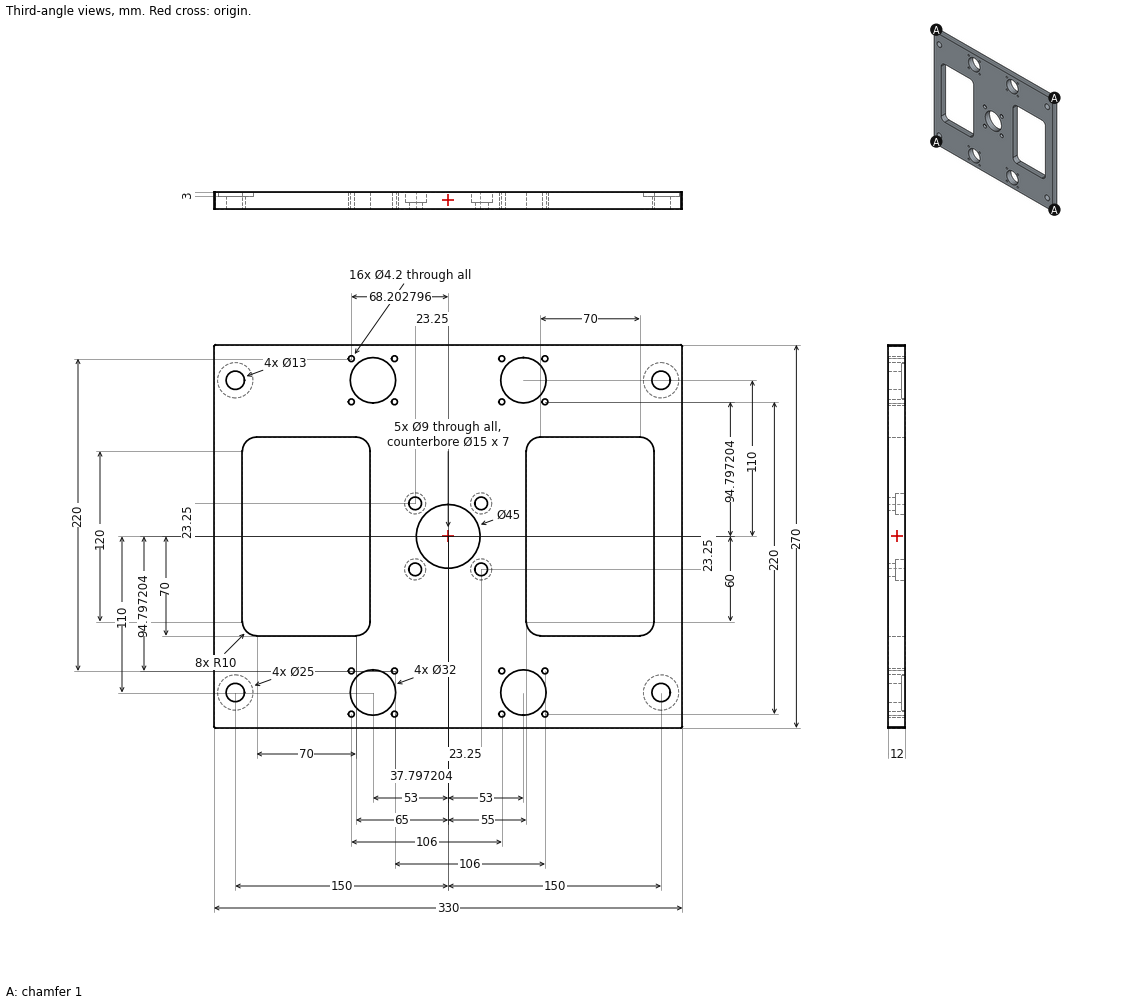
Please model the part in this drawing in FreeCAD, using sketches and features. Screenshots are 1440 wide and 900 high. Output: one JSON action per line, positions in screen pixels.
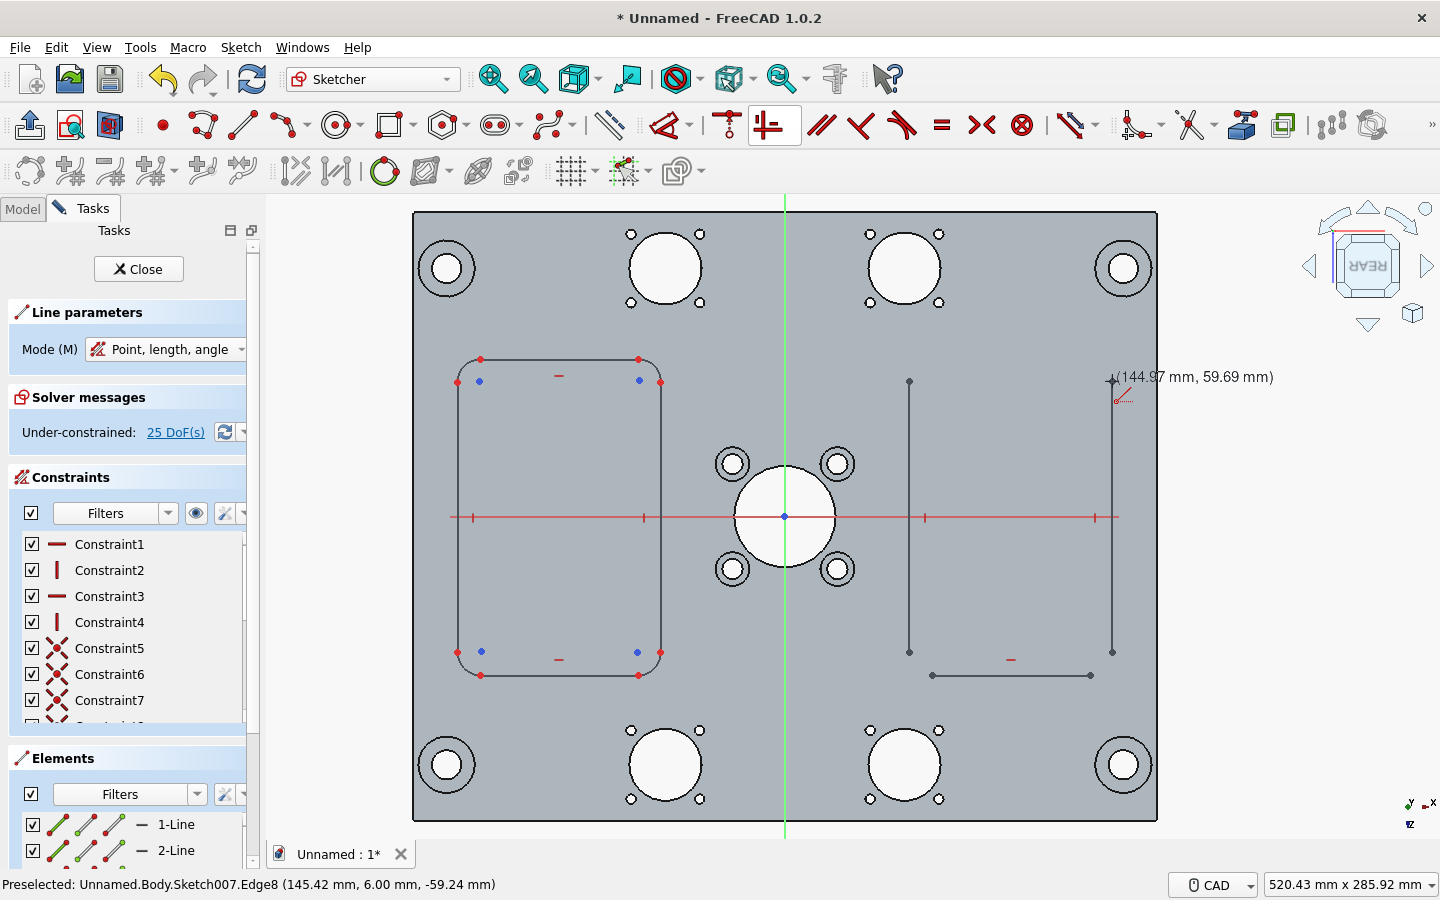
{"action": "left_click", "coordinate": [1090, 359]}
{"action": "left_click", "coordinate": [932, 359]}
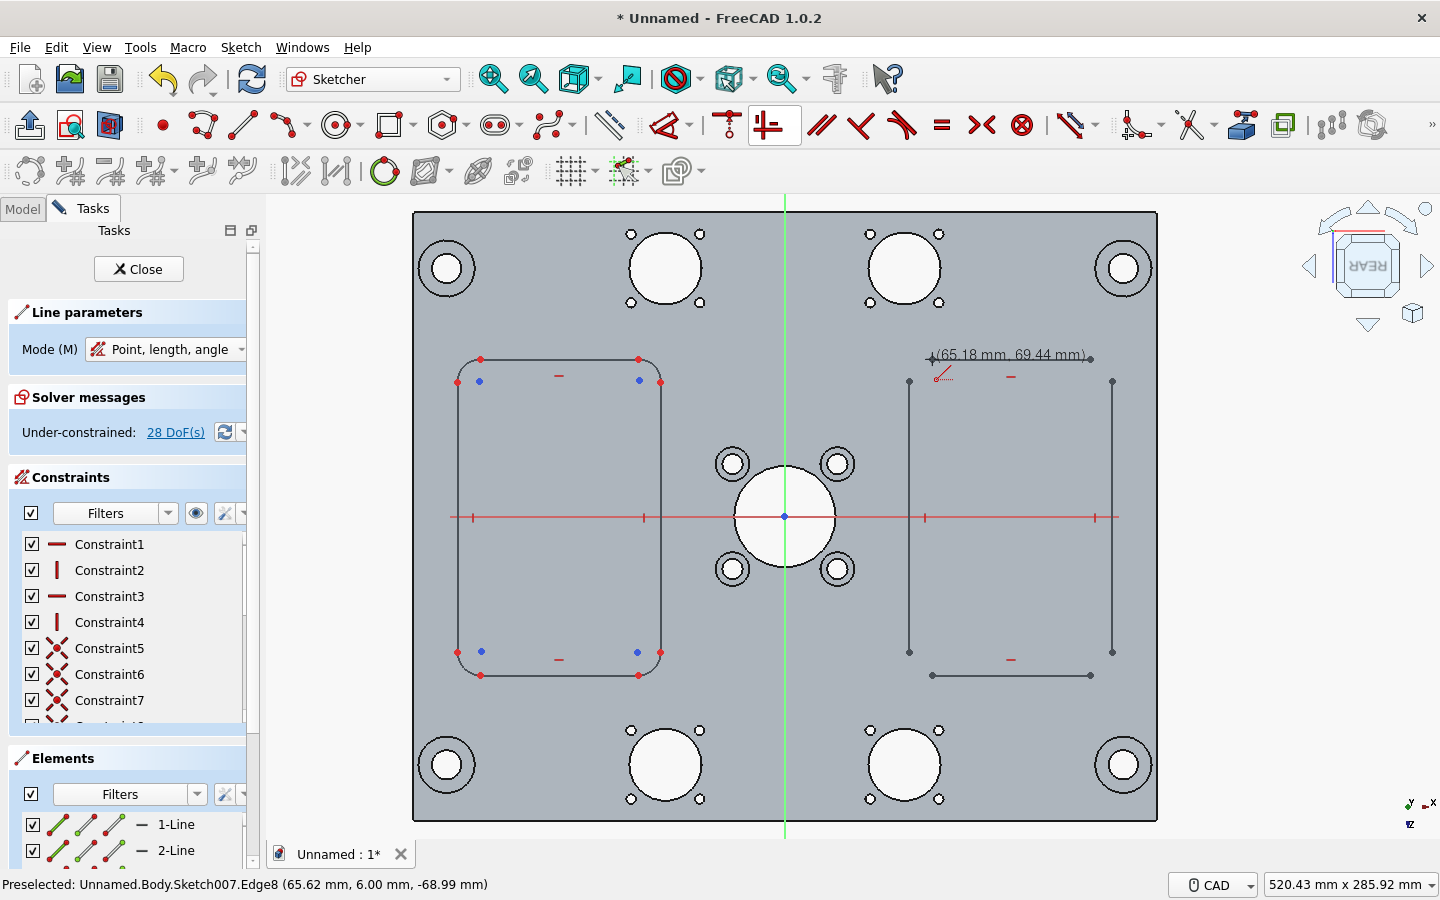
{"action": "left_click", "coordinate": [284, 126]}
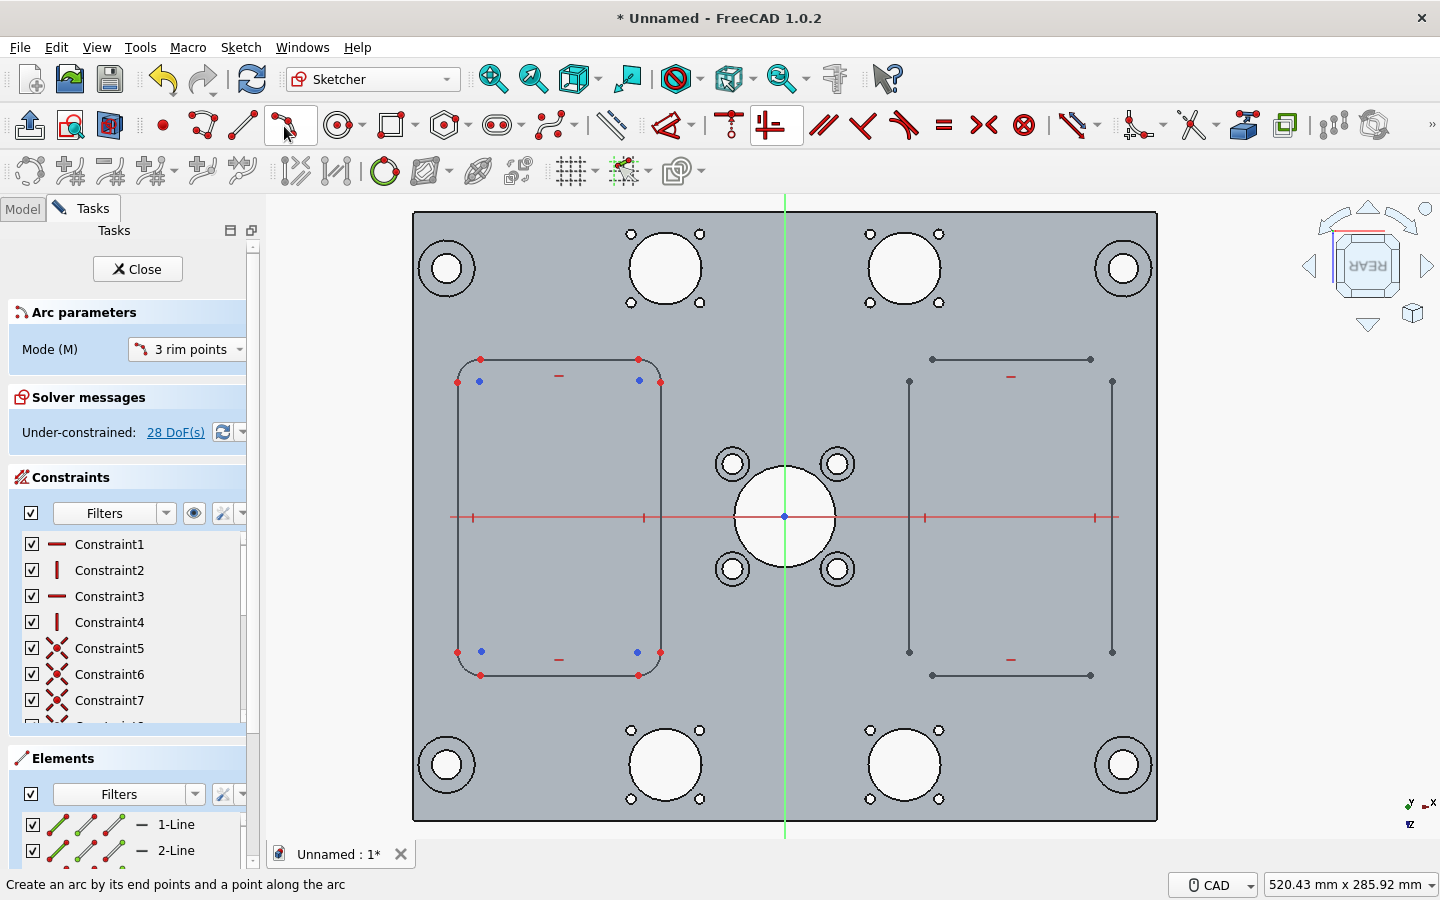
{"action": "left_click", "coordinate": [909, 653]}
{"action": "left_click", "coordinate": [932, 676]}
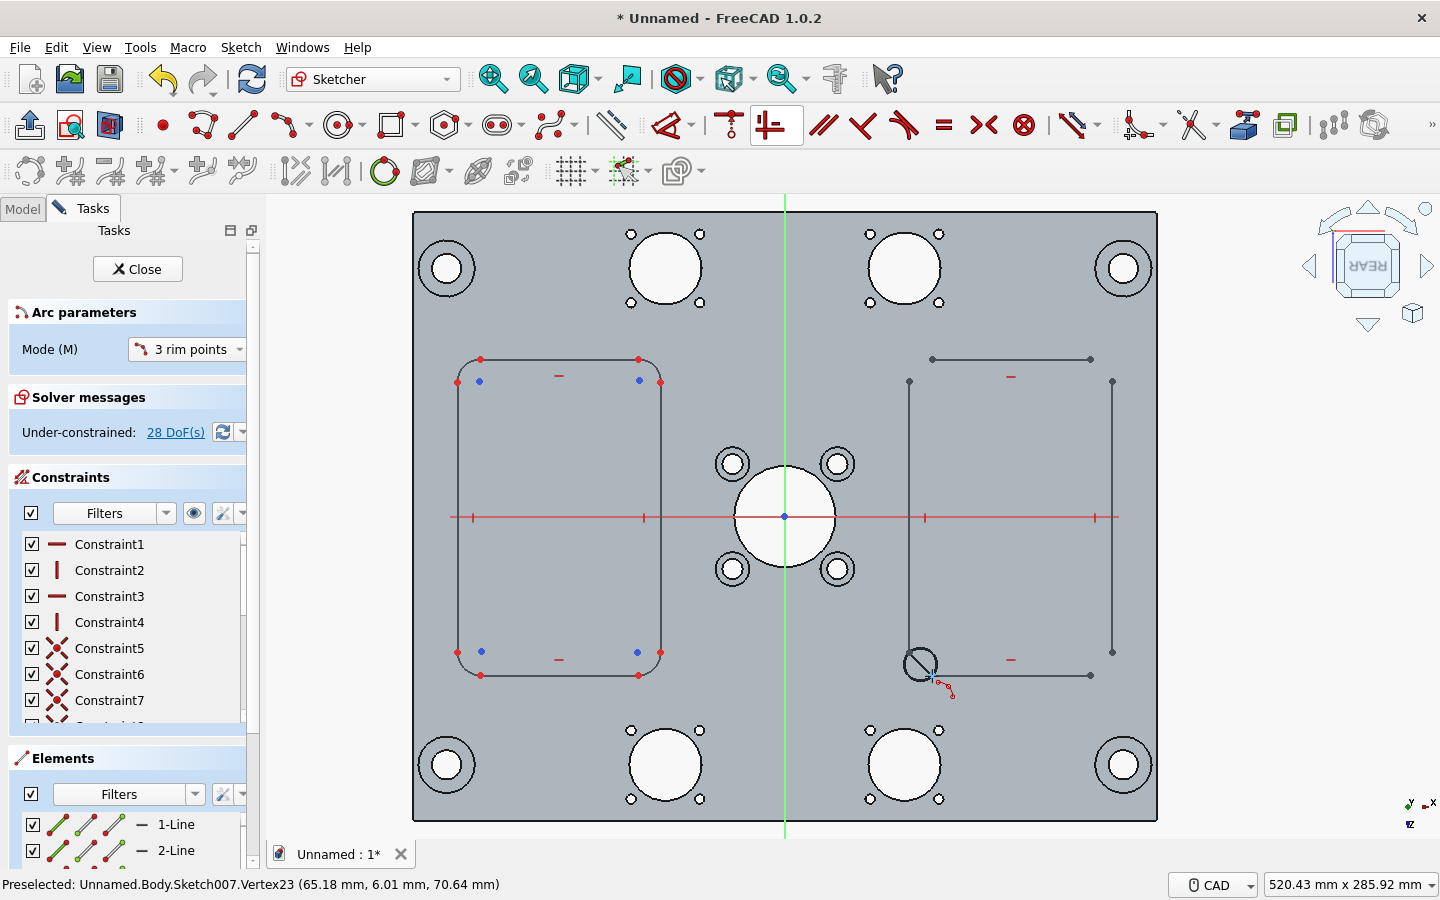
{"action": "scroll", "coordinate": [916, 668], "scroll_direction": "up", "scroll_amount": 5}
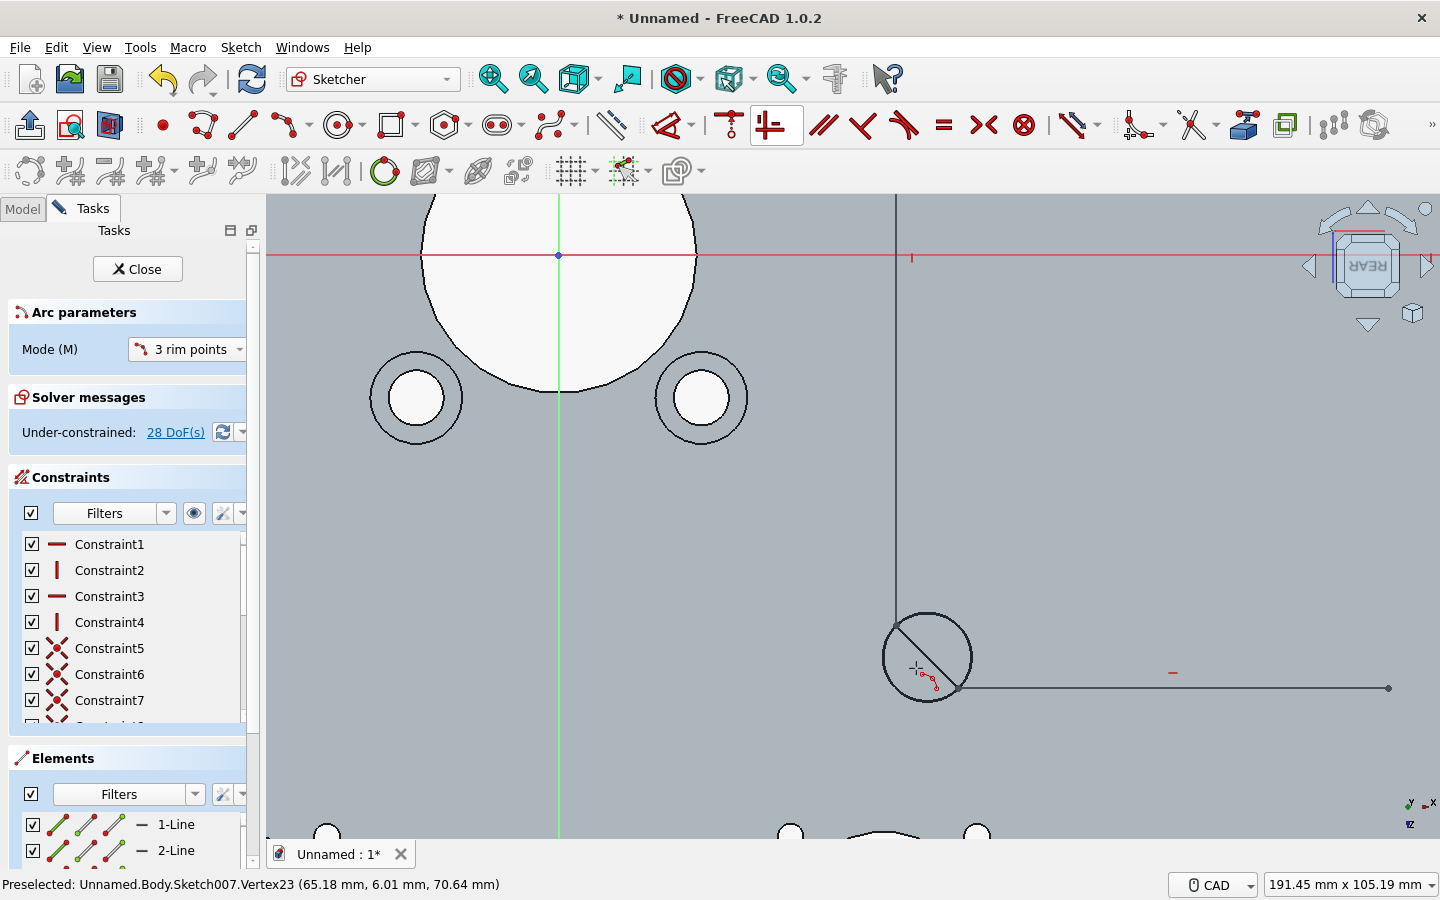
{"action": "left_click", "coordinate": [914, 667]}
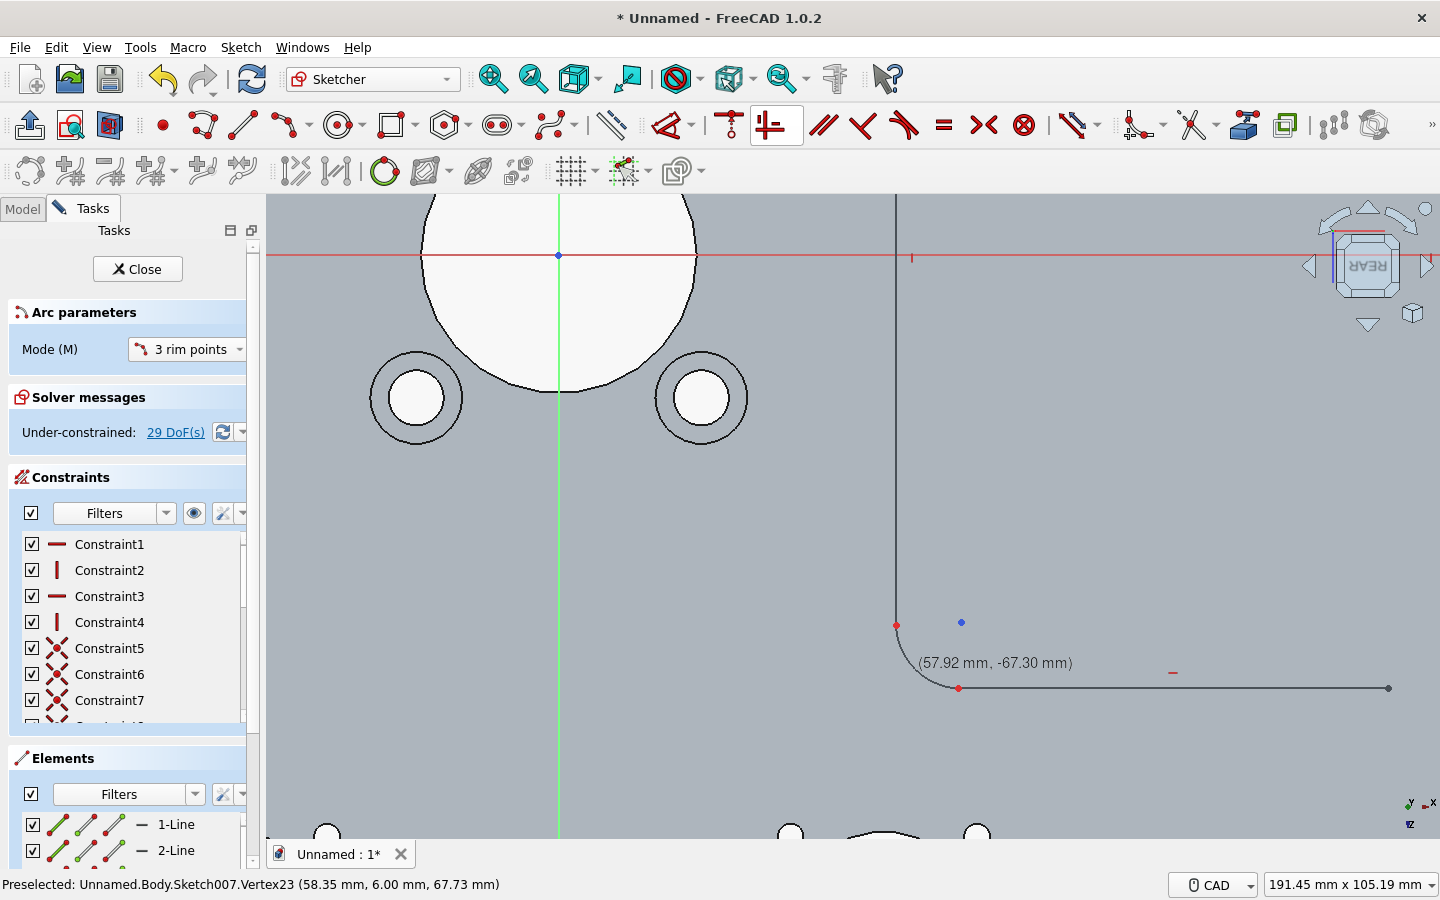
{"action": "scroll", "coordinate": [916, 669], "scroll_direction": "down", "scroll_amount": 5}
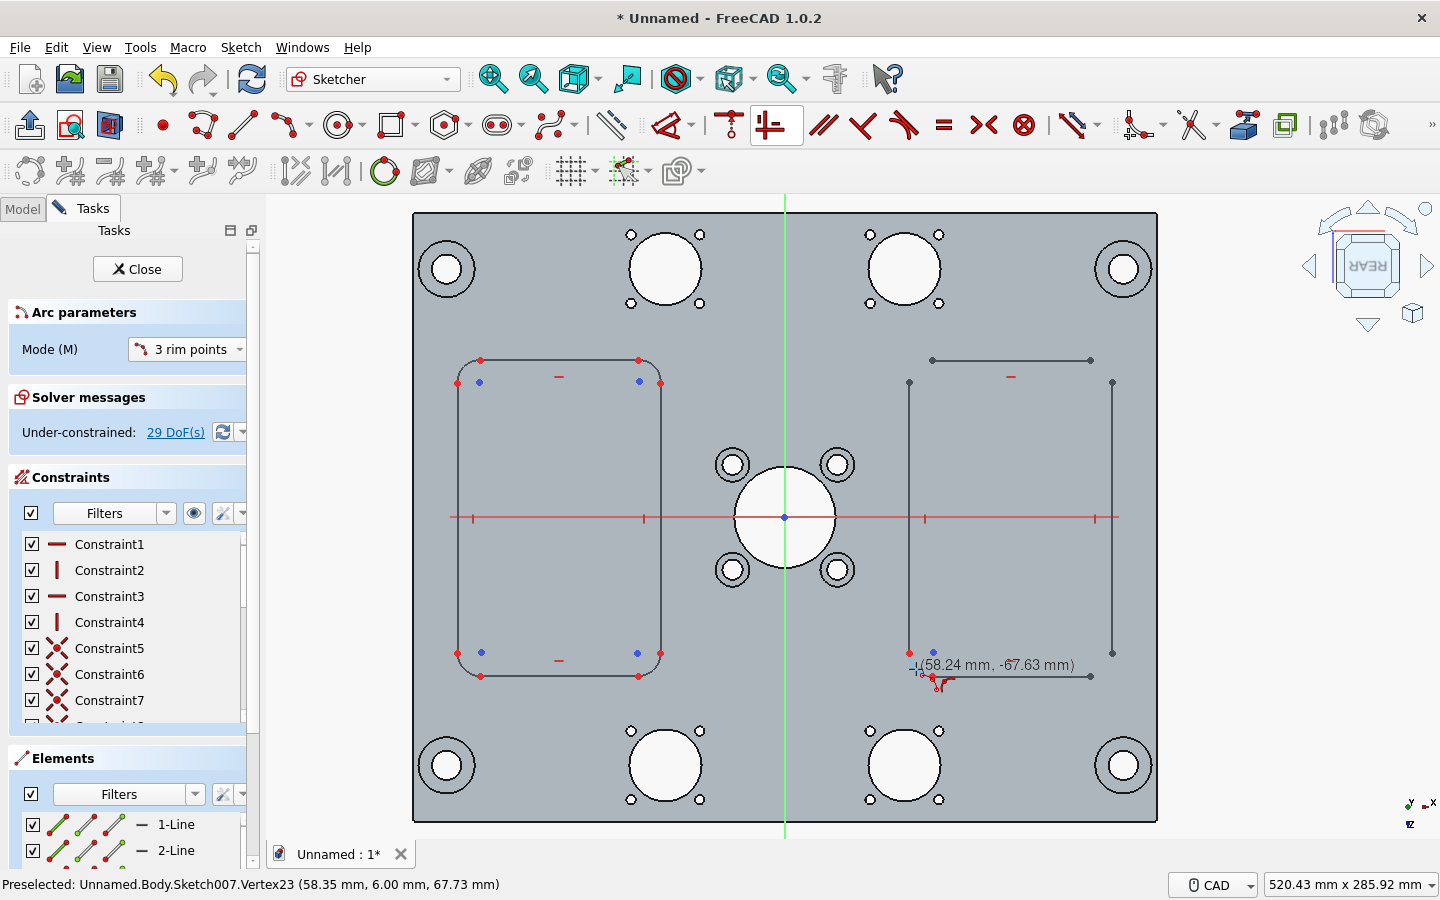
{"action": "left_click", "coordinate": [1090, 677]}
{"action": "left_click", "coordinate": [1112, 654]}